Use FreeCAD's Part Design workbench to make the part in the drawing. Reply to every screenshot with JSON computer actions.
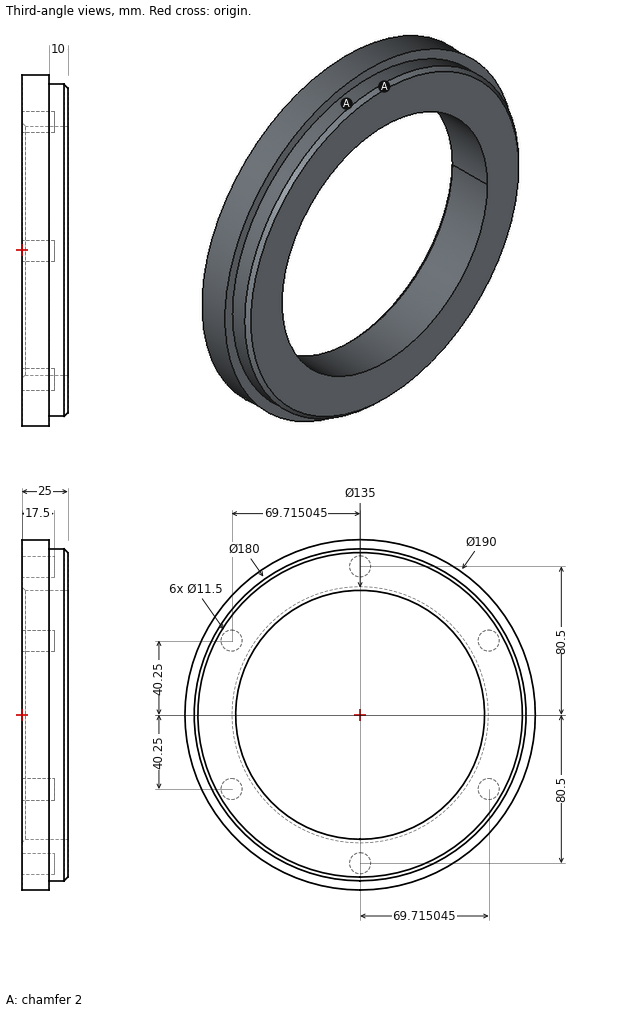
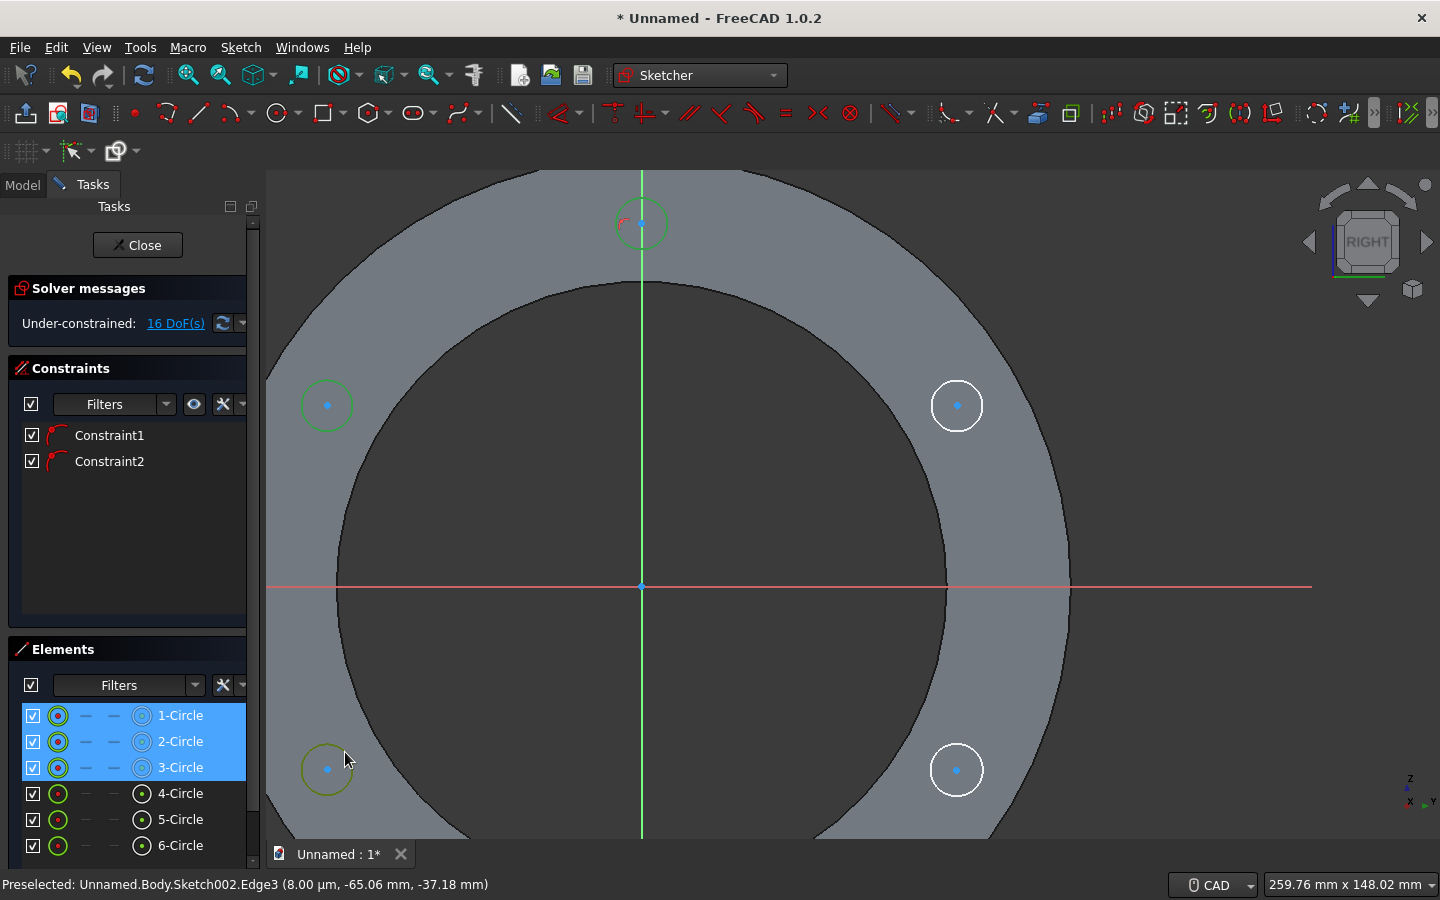
{"action": "scroll", "coordinate": [958, 404], "scroll_direction": "down", "scroll_amount": 3}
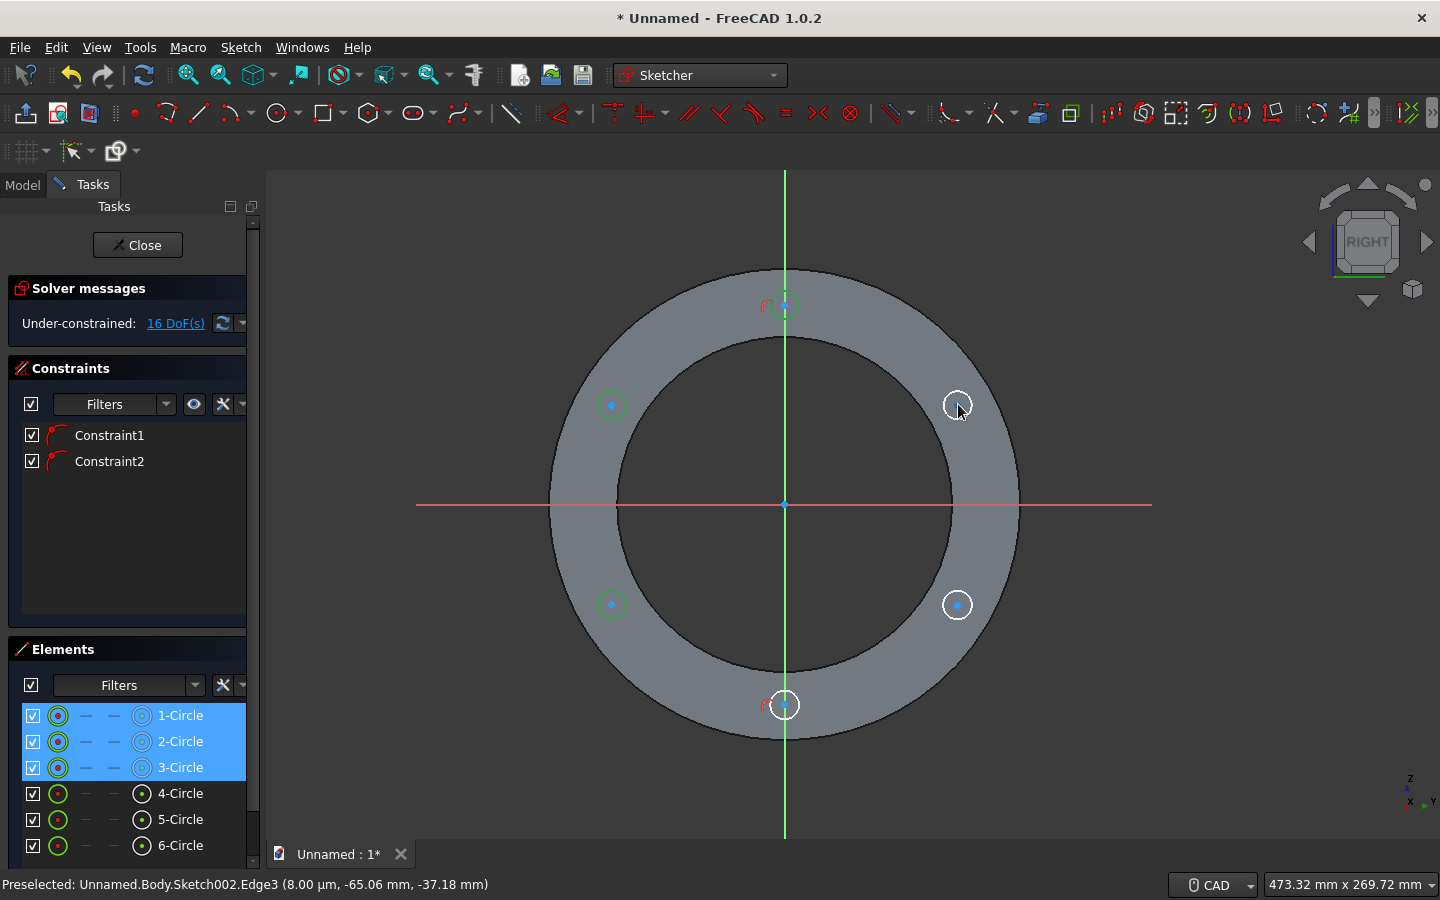
{"action": "scroll", "coordinate": [795, 695], "scroll_direction": "up", "scroll_amount": 2}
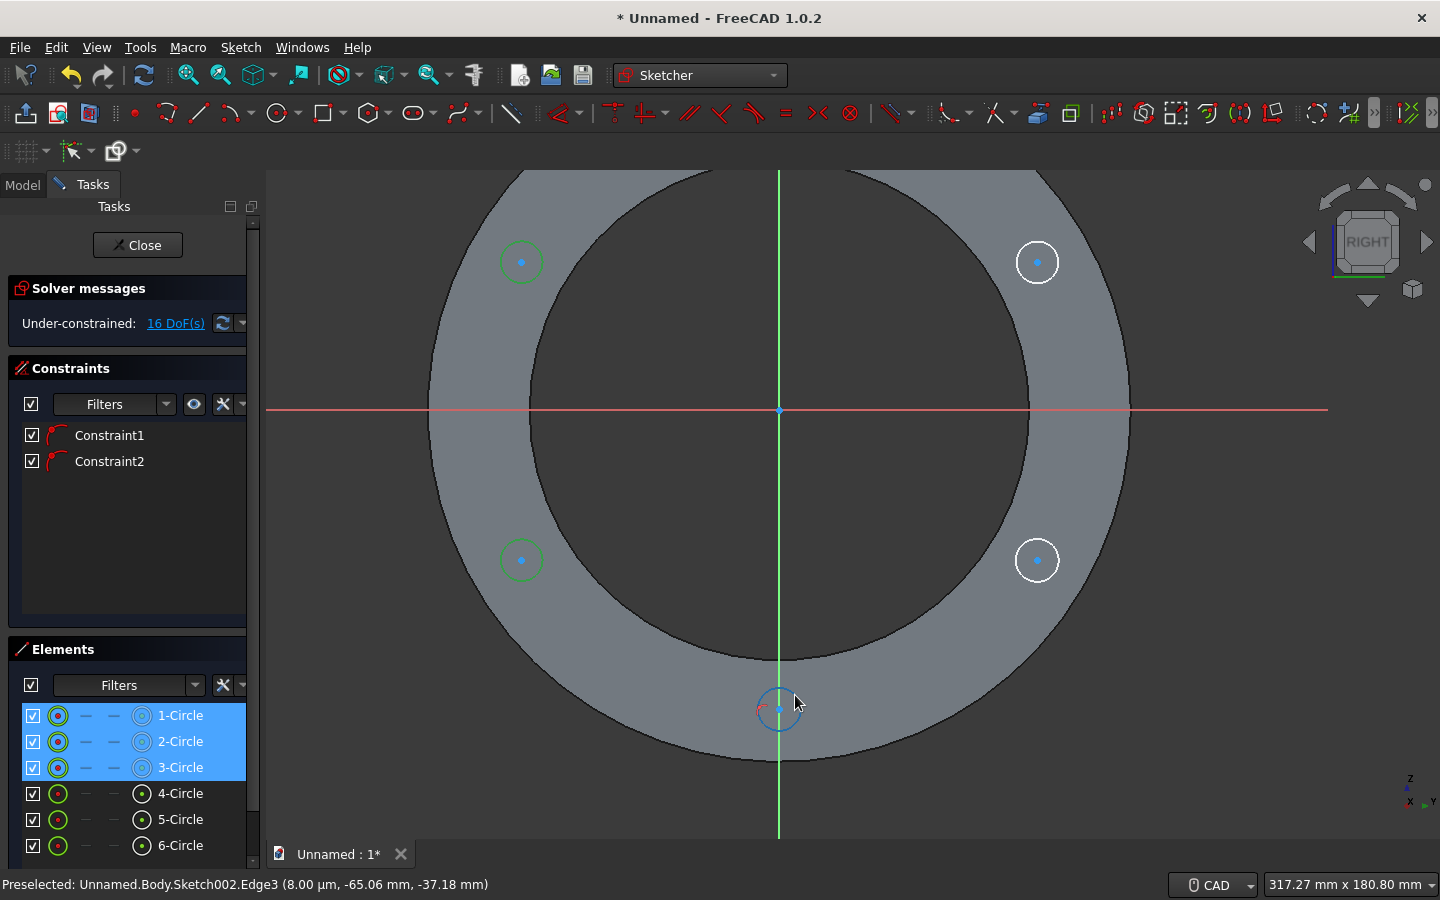
{"action": "left_click", "coordinate": [794, 694]}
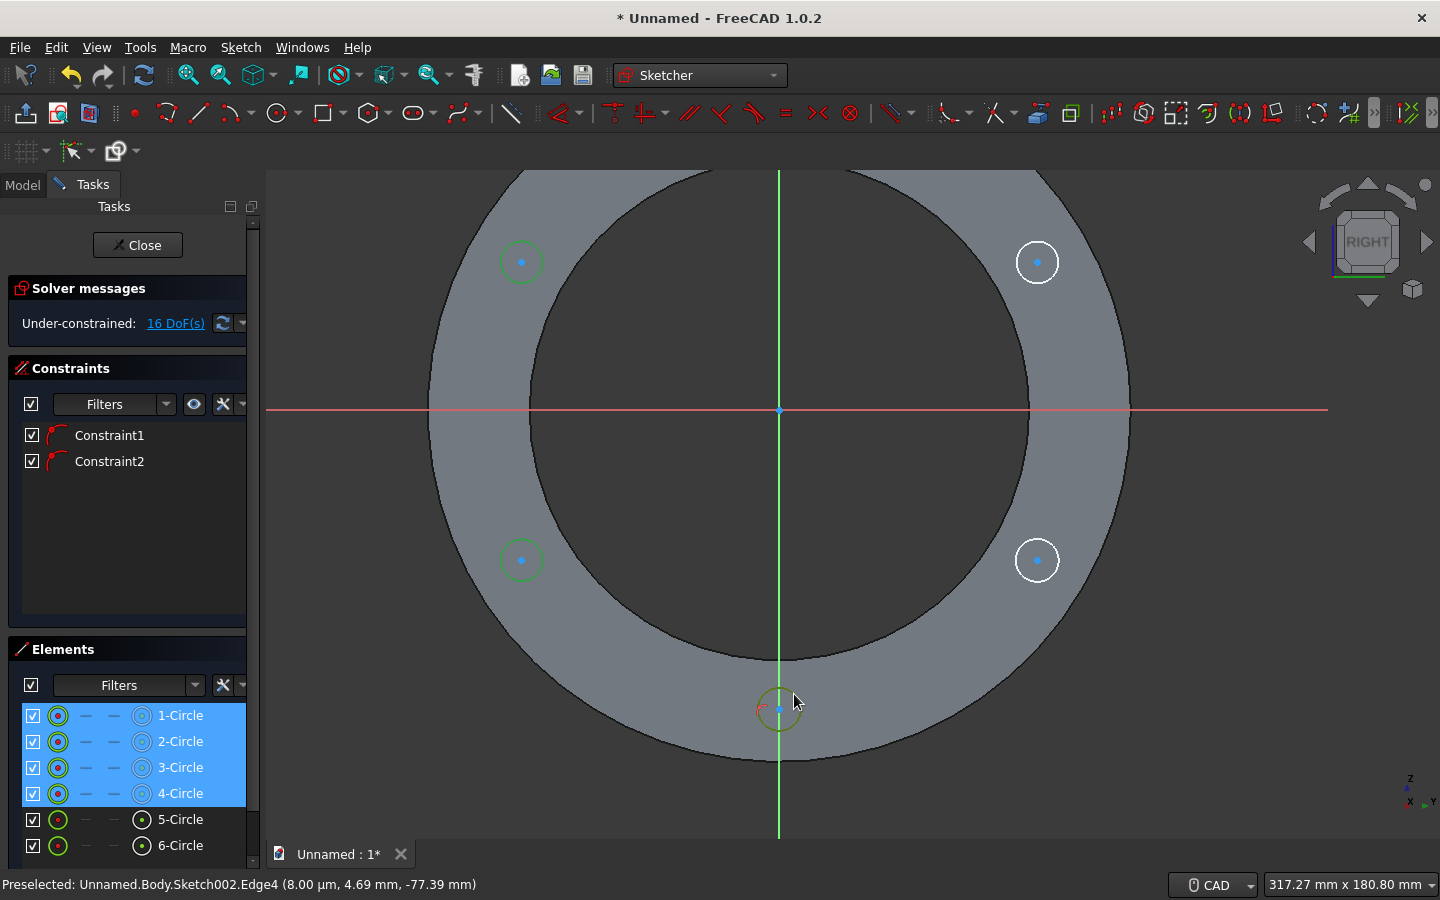
{"action": "left_click", "coordinate": [1052, 545]}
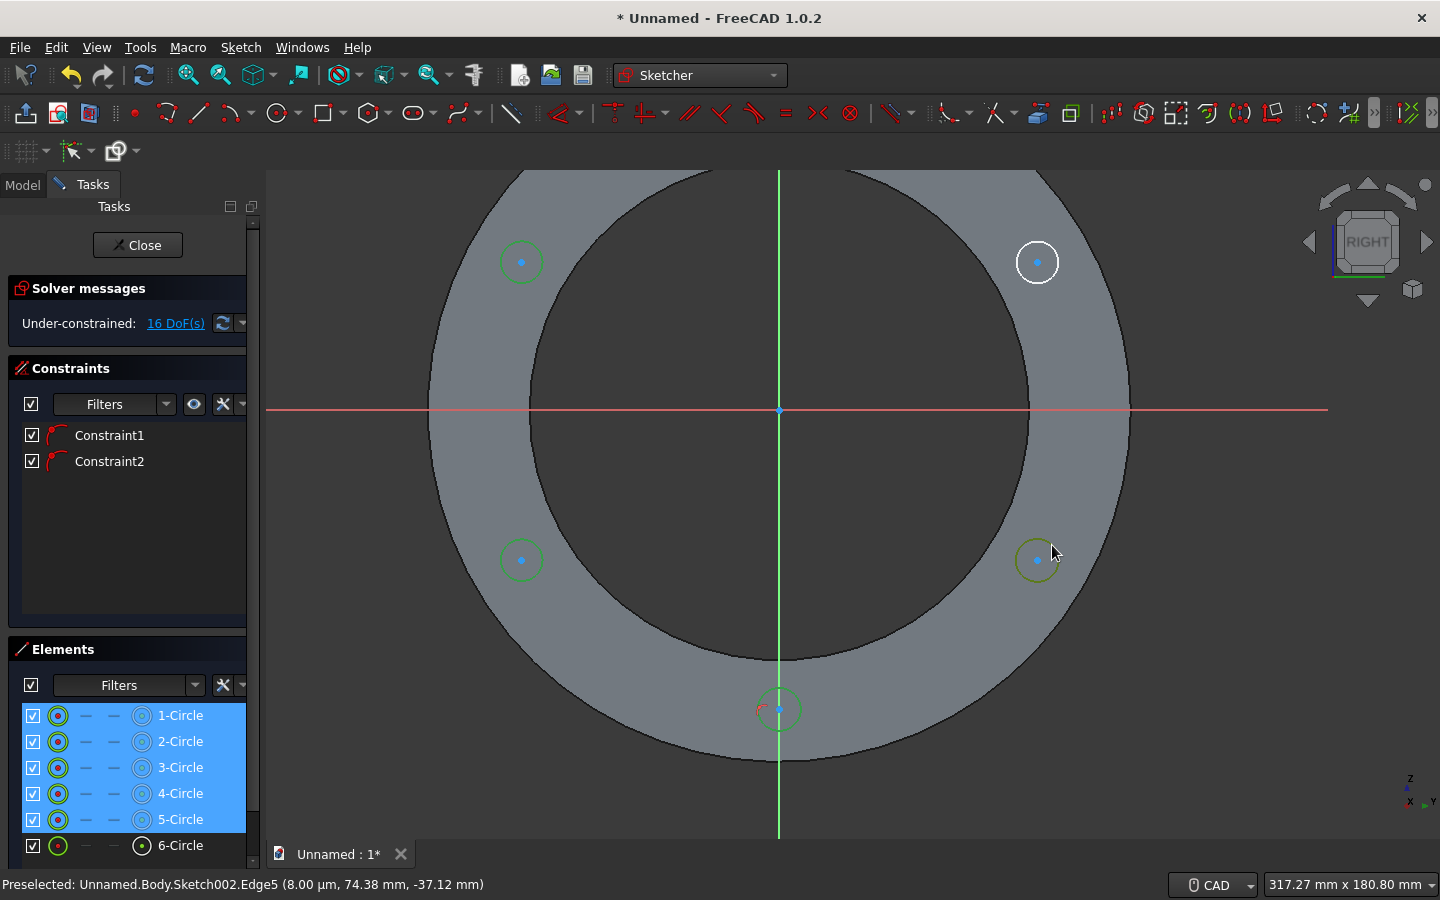
{"action": "left_click", "coordinate": [1052, 248]}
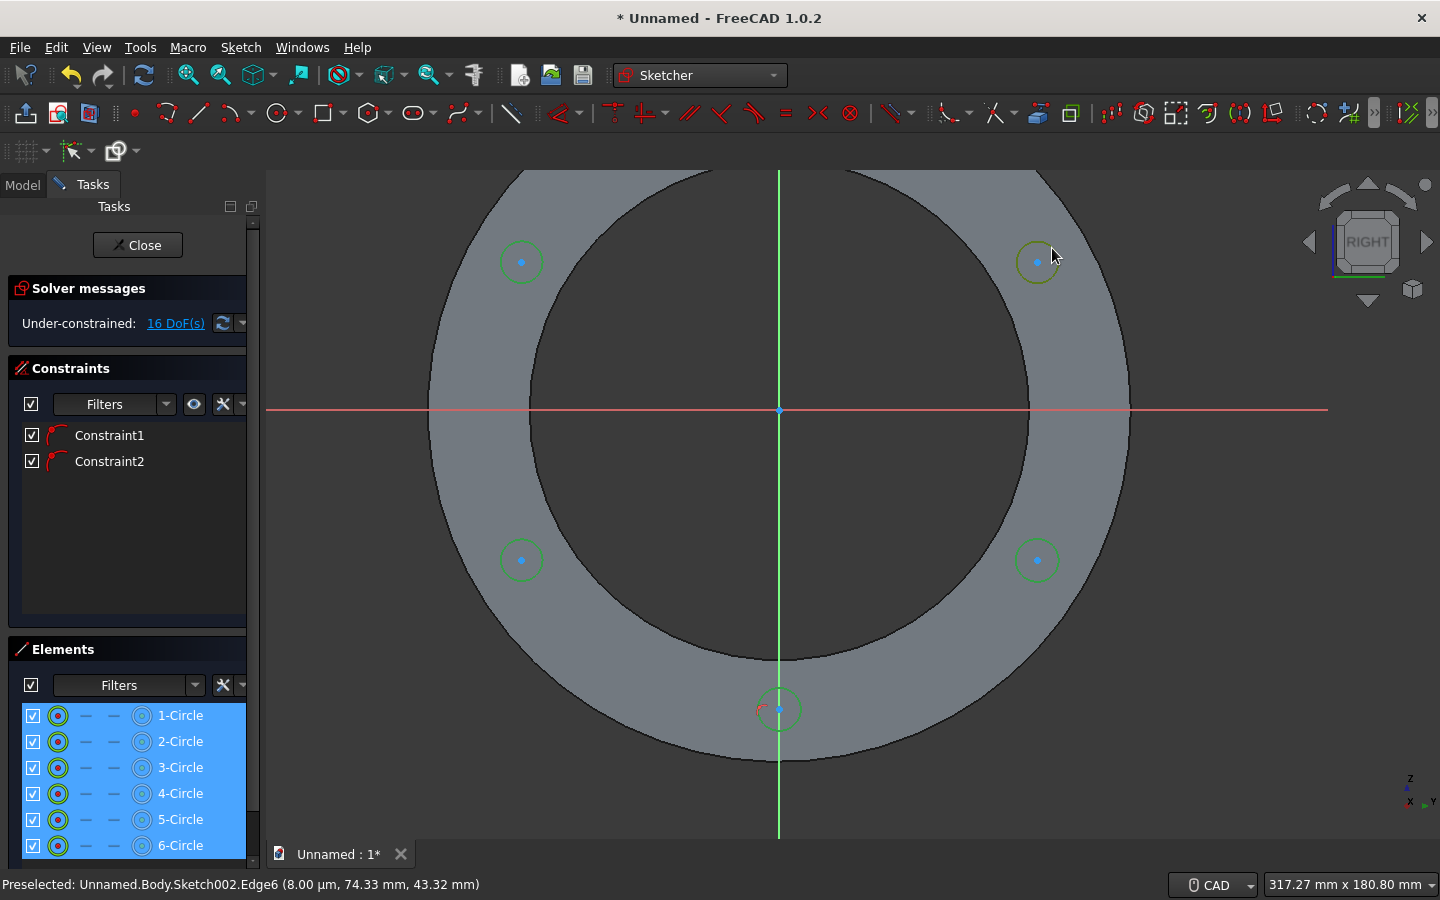
{"action": "left_click", "coordinate": [786, 114]}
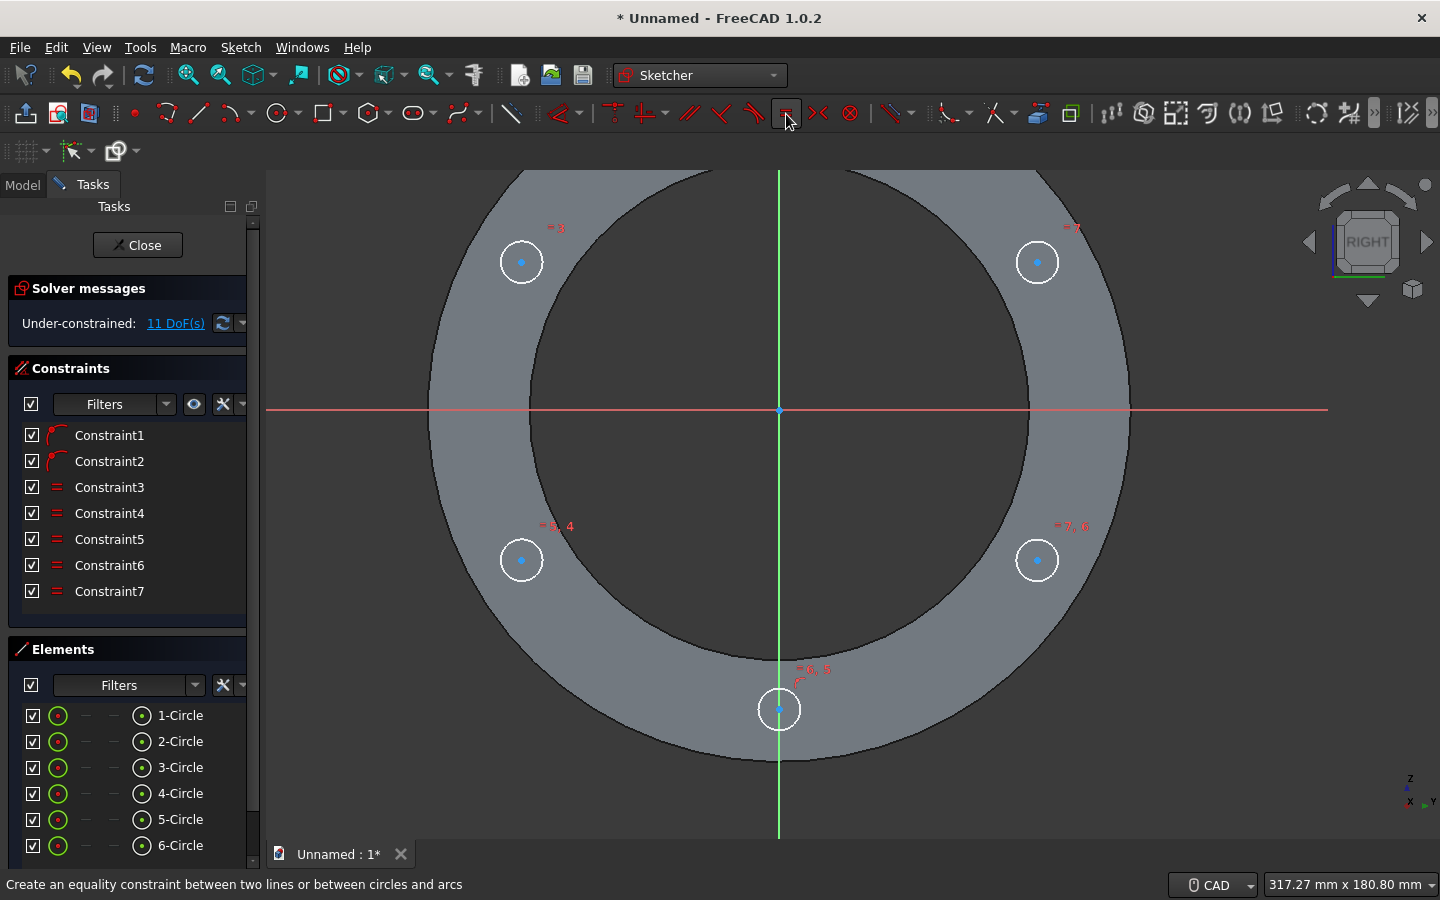
{"action": "left_click", "coordinate": [522, 262]}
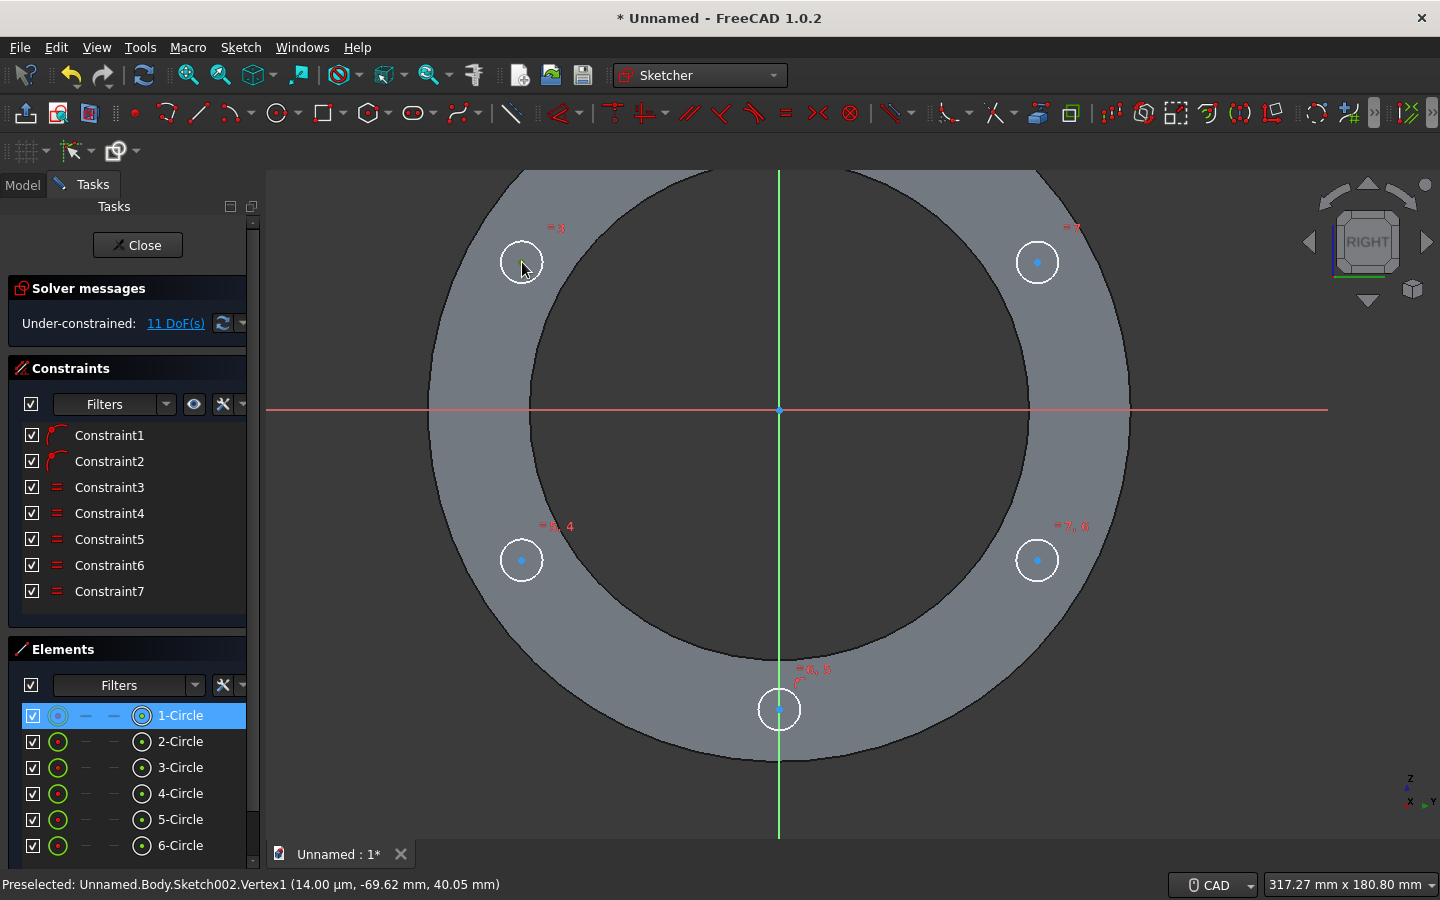
{"action": "left_click", "coordinate": [522, 560]}